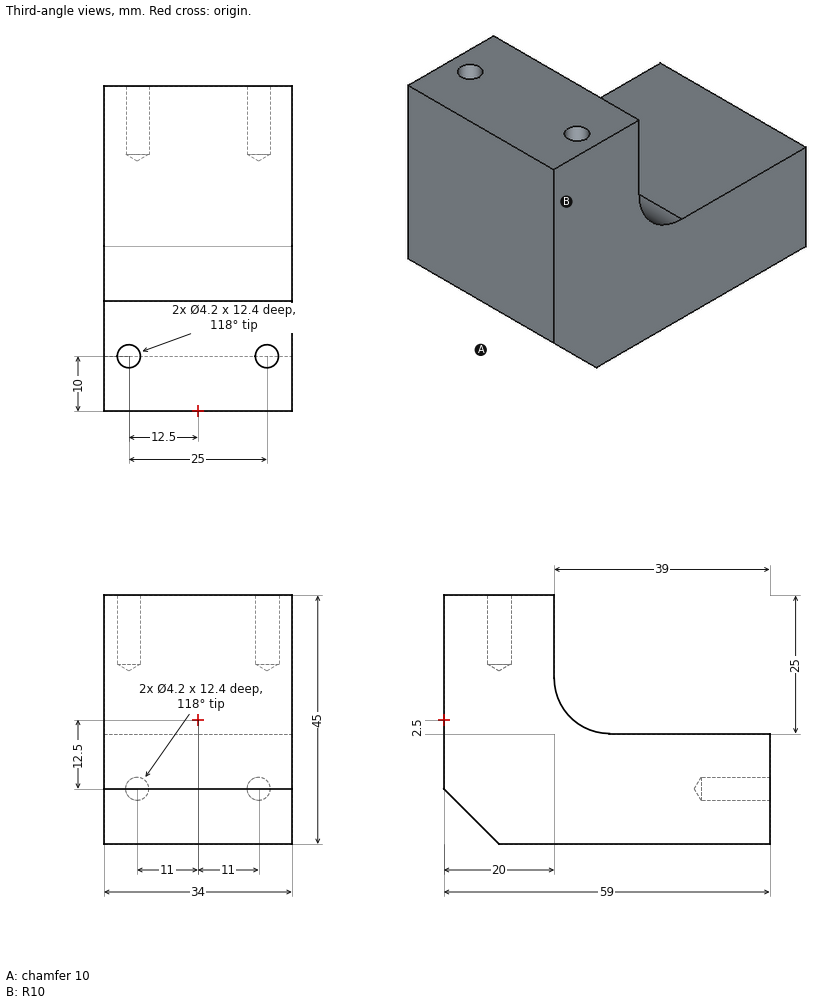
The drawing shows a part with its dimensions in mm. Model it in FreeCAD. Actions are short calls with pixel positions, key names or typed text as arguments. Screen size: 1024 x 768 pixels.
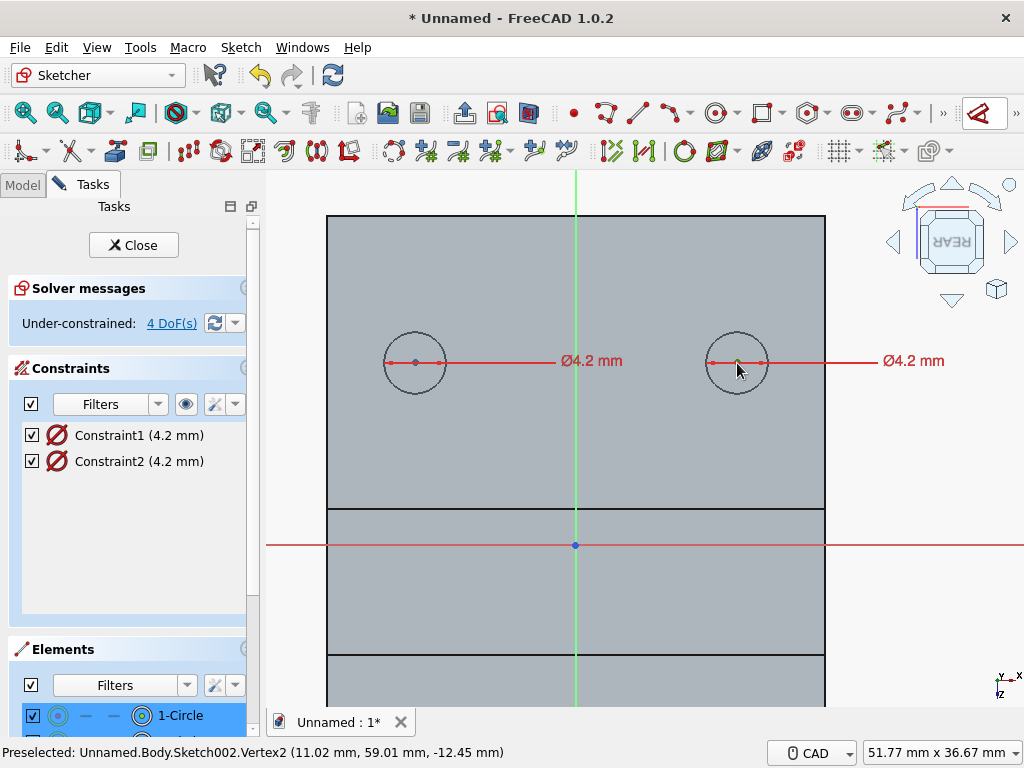
key(h)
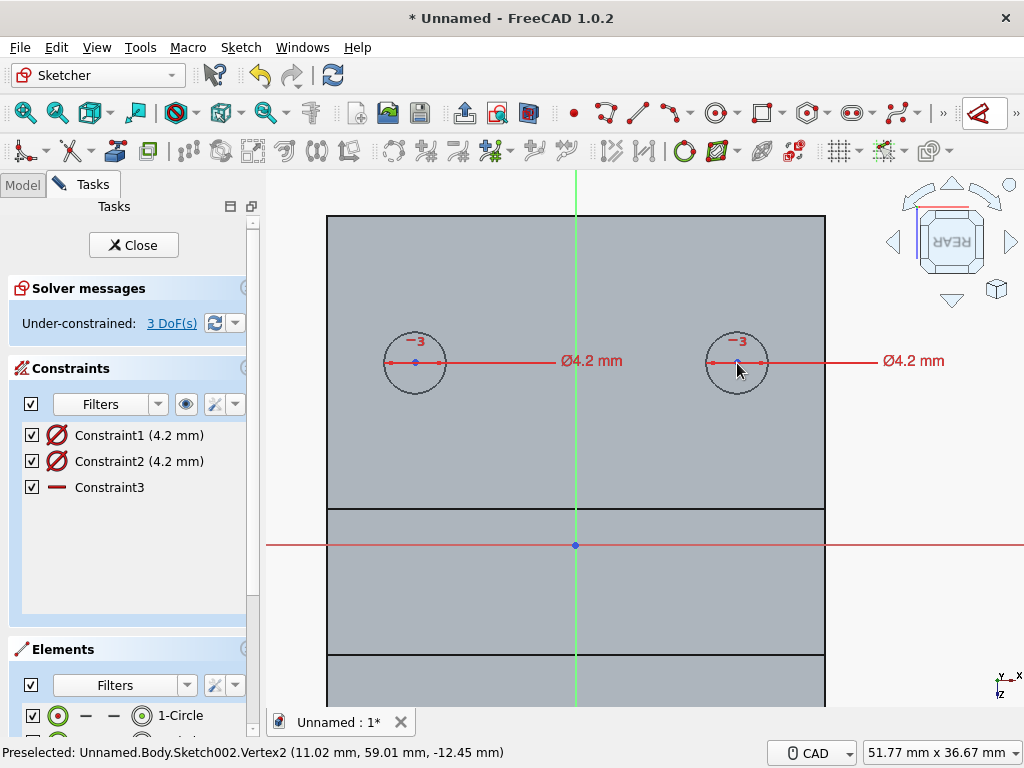
click(415, 363)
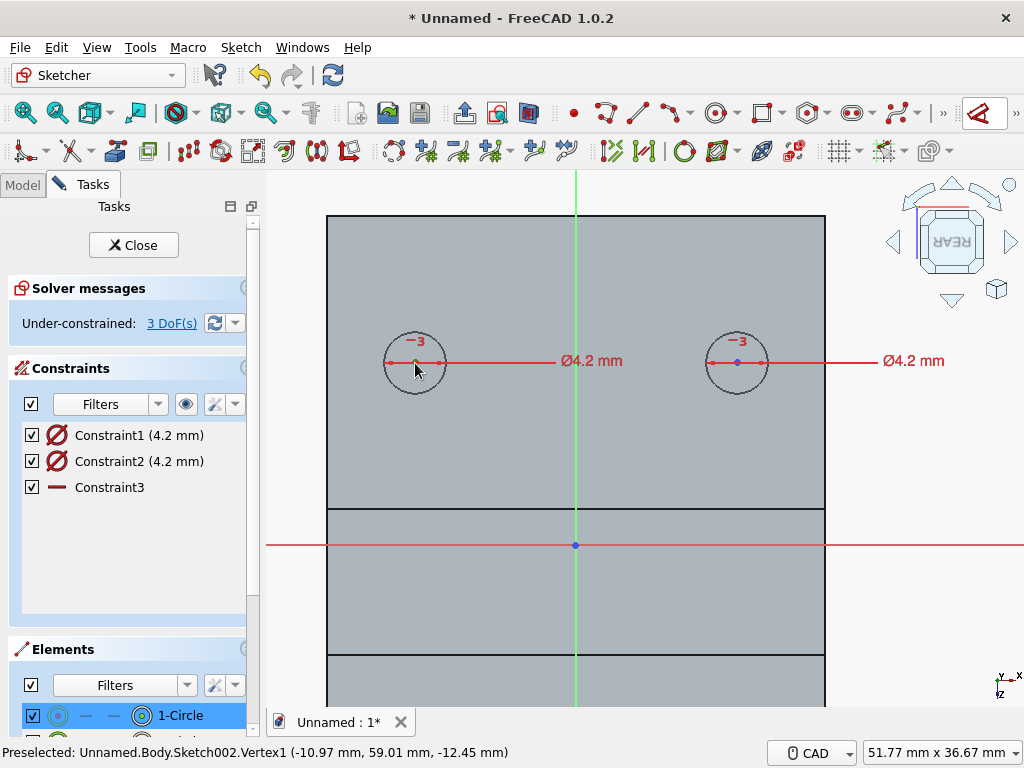
click(1002, 114)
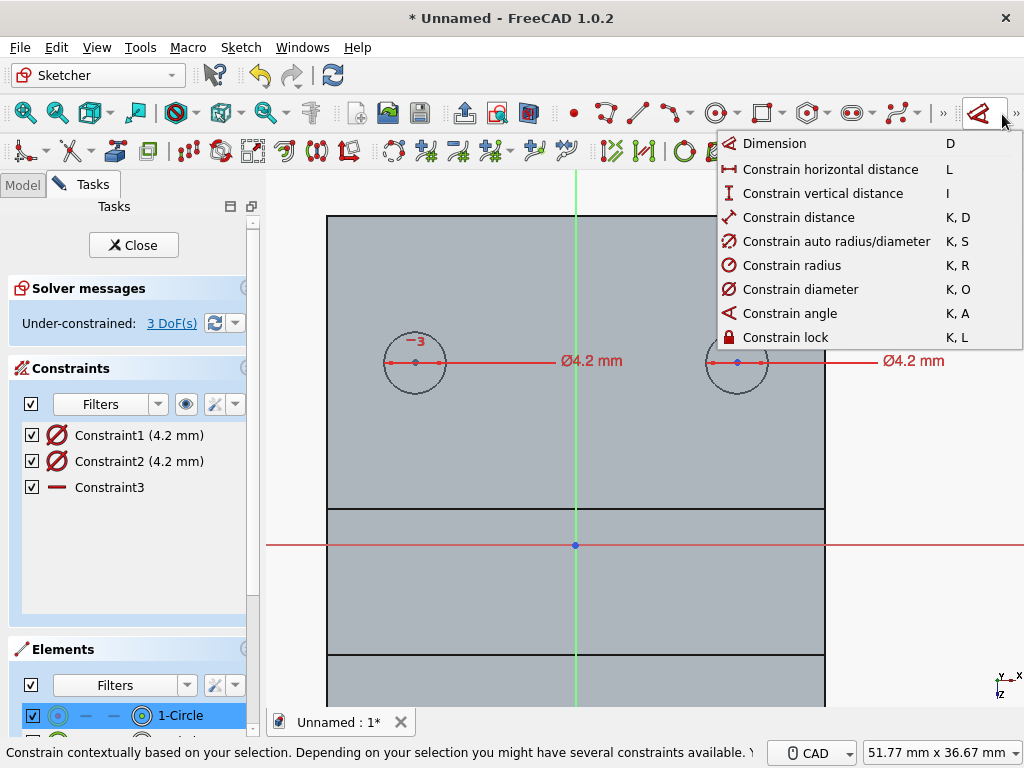
click(870, 169)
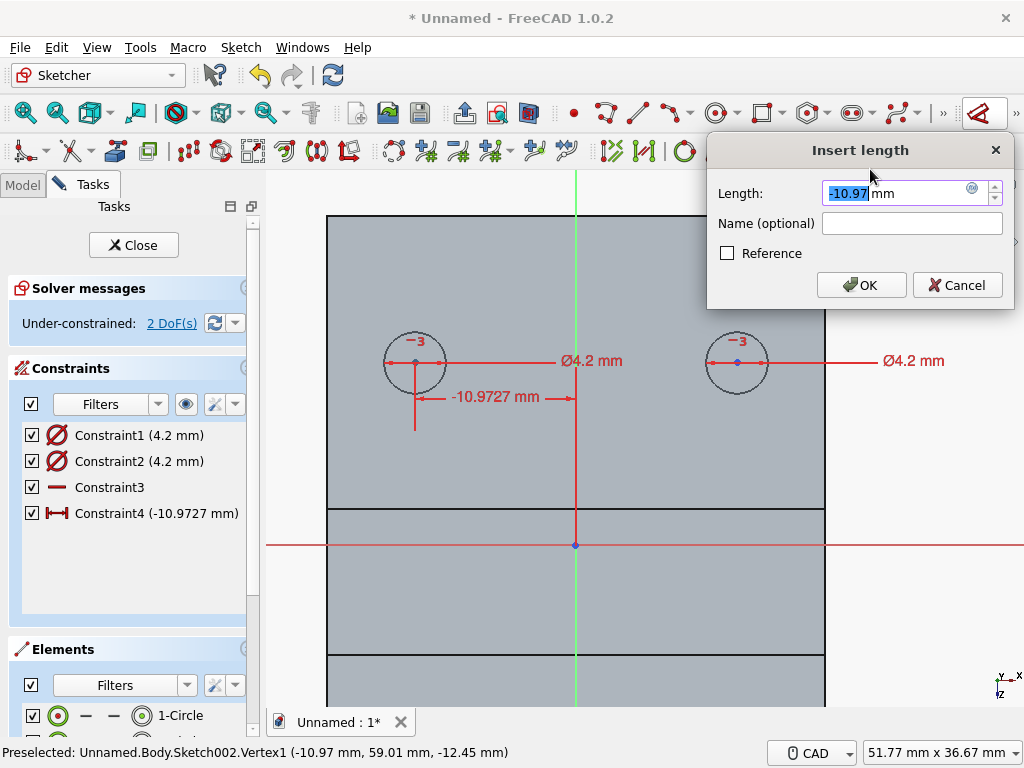
text(-11)
key(Return)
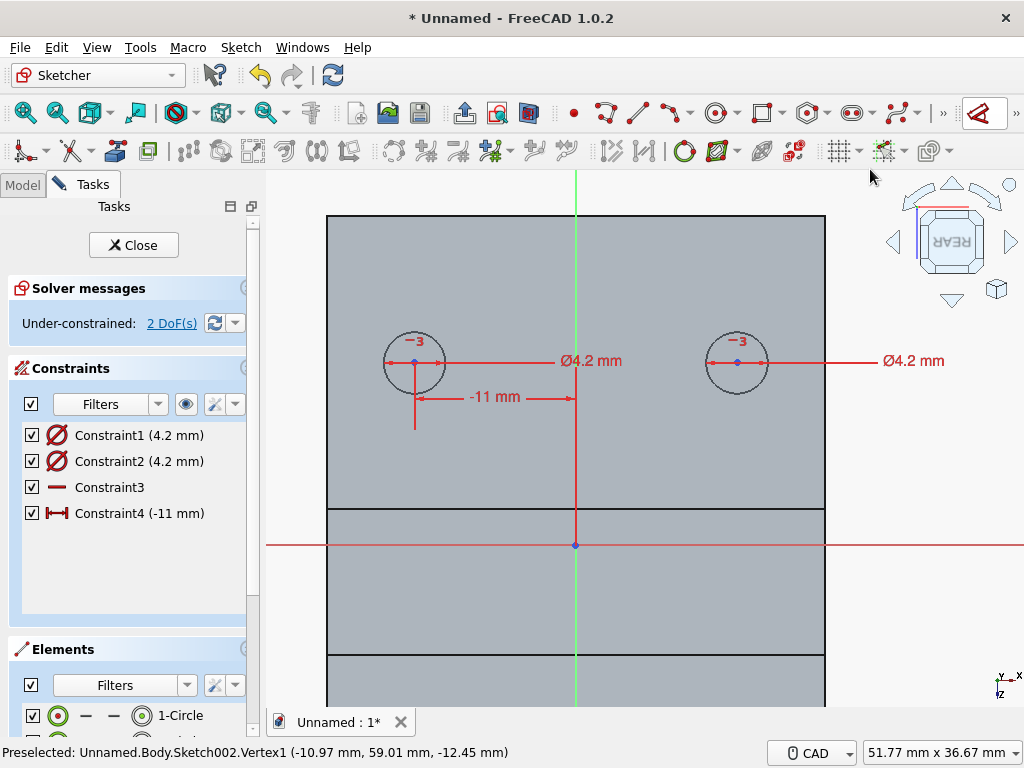
click(737, 363)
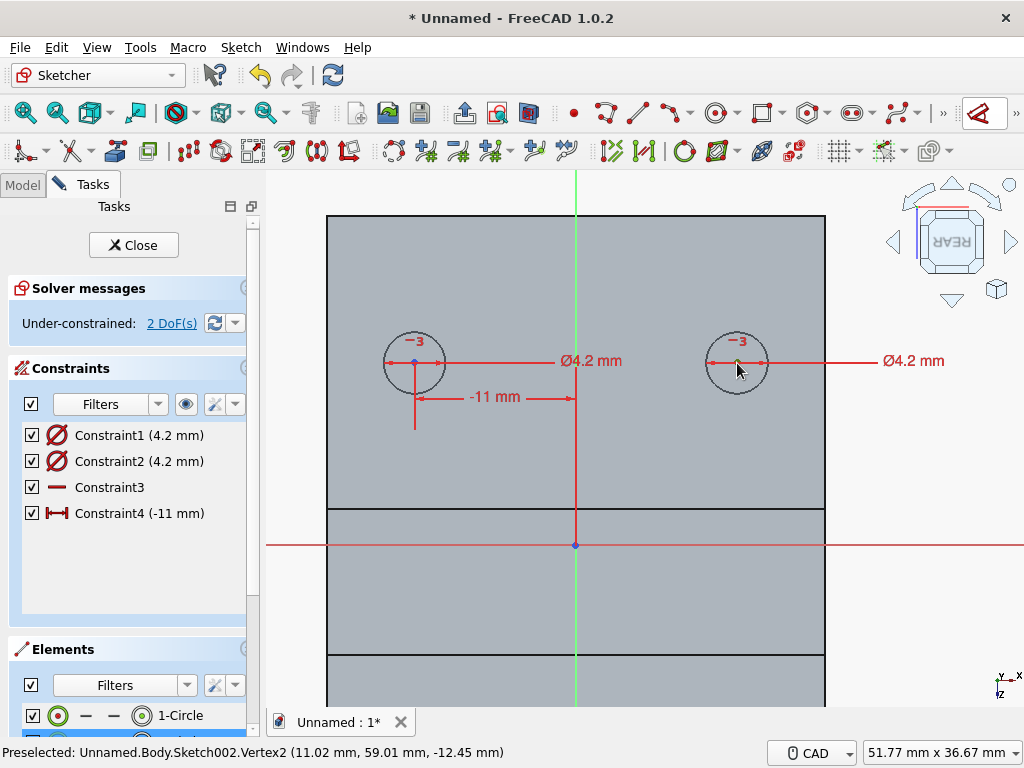
key(l)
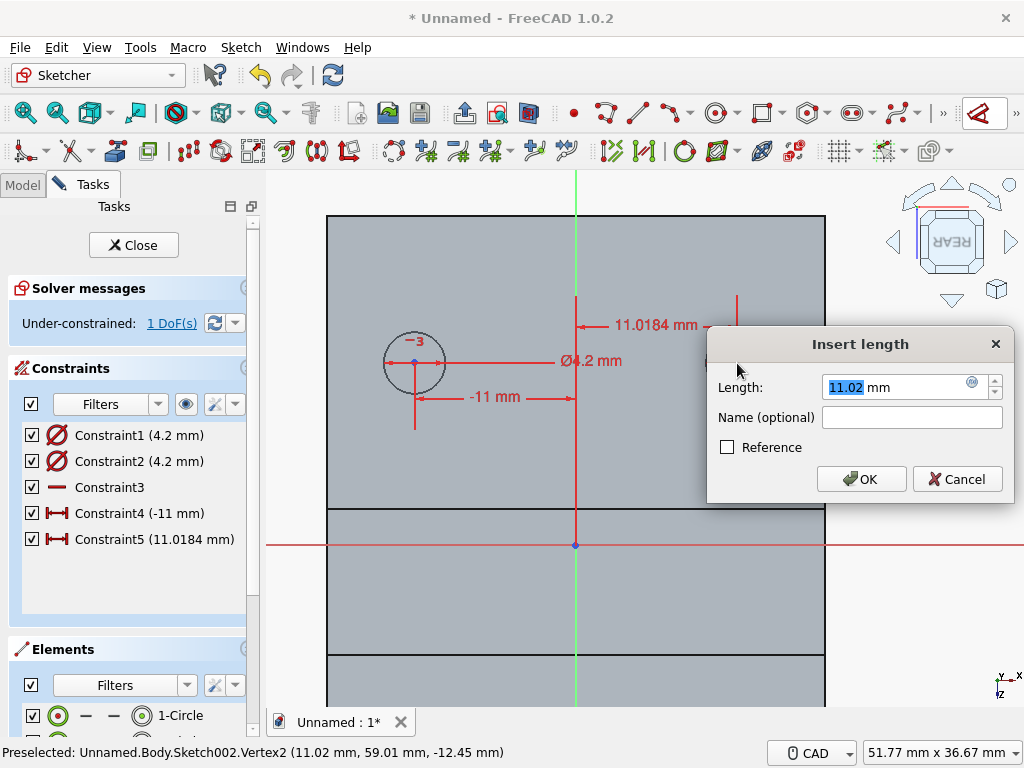
text(11)
key(Return)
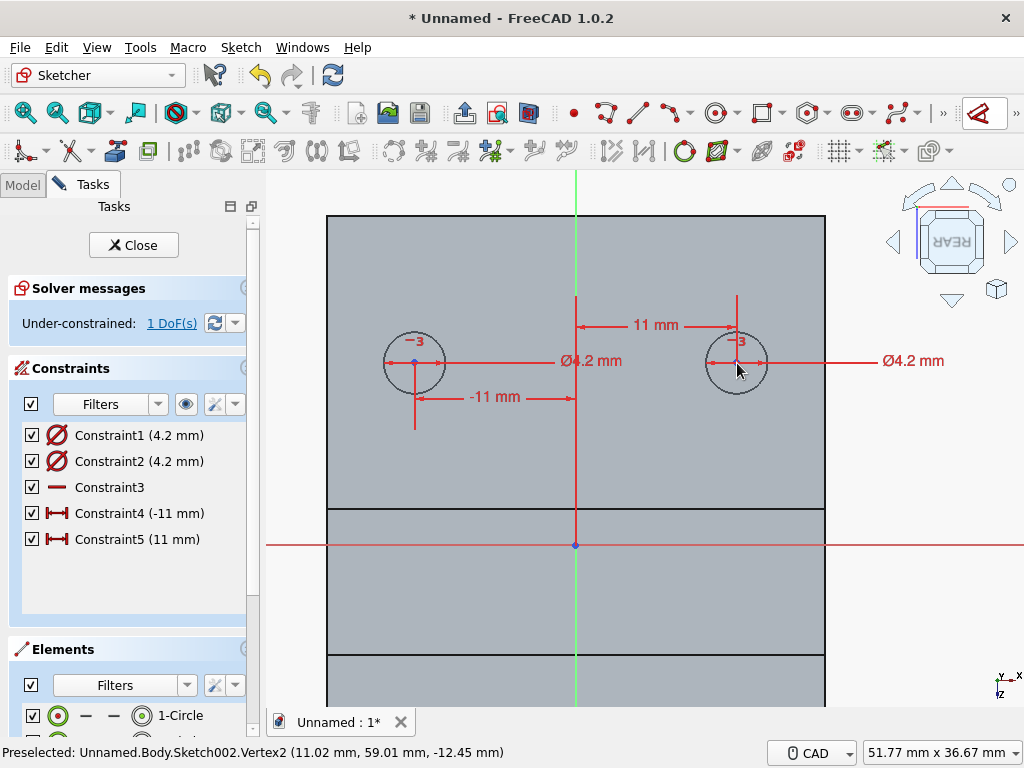
click(415, 363)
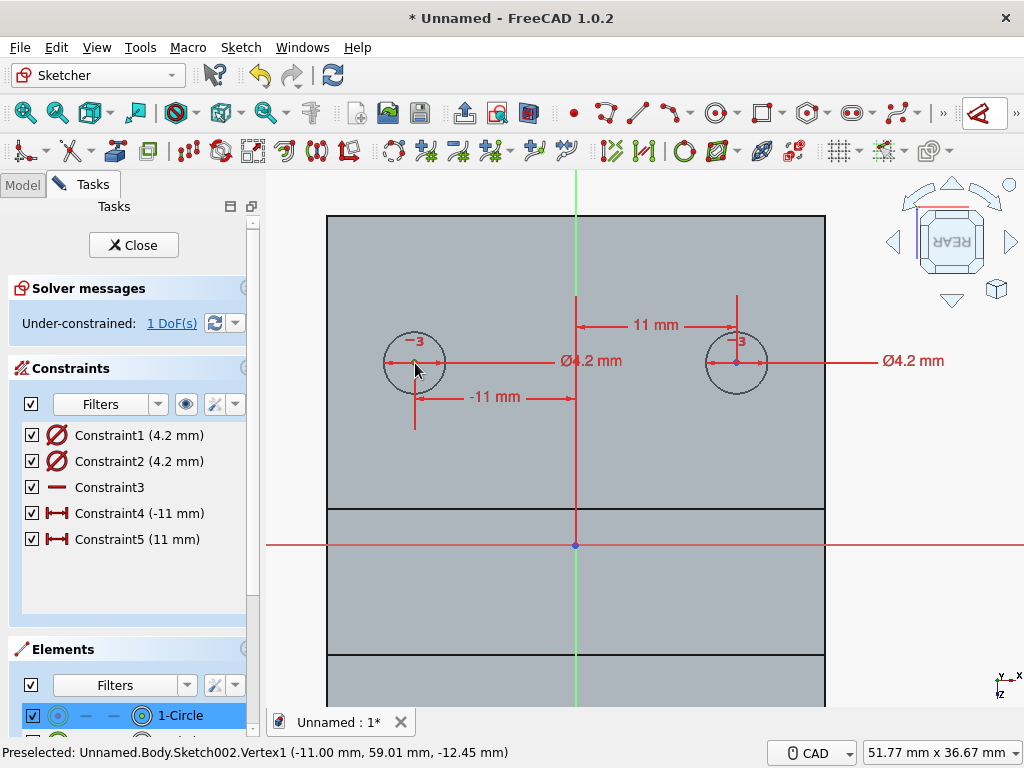
key(i)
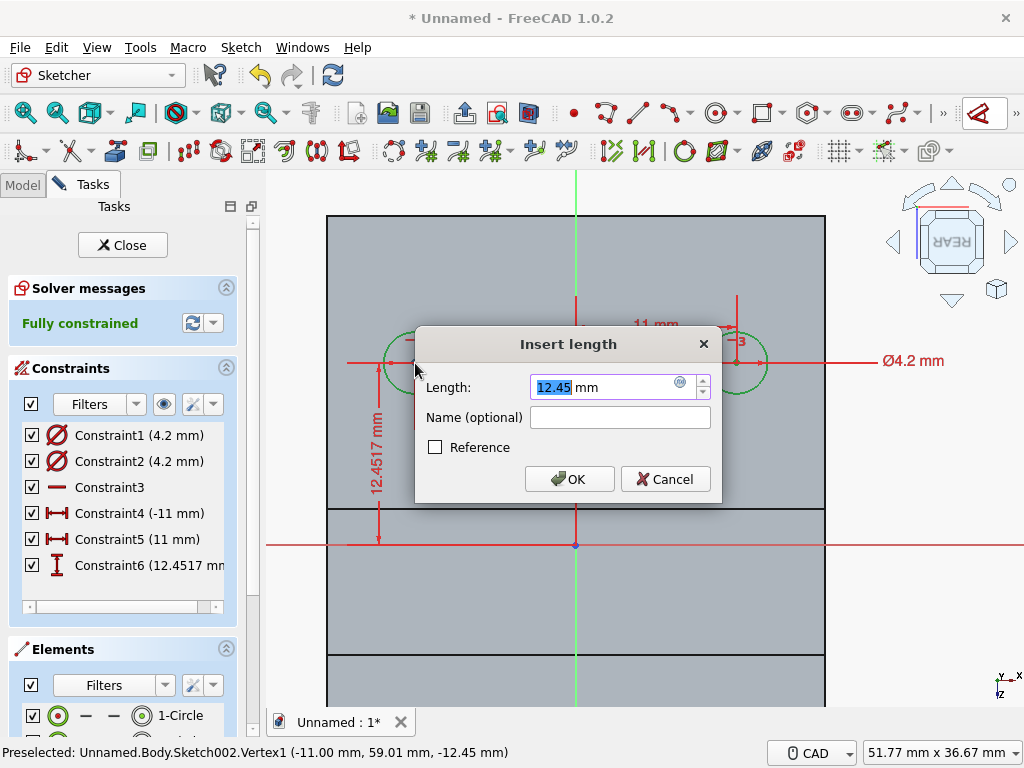
text(12.5)
key(Return)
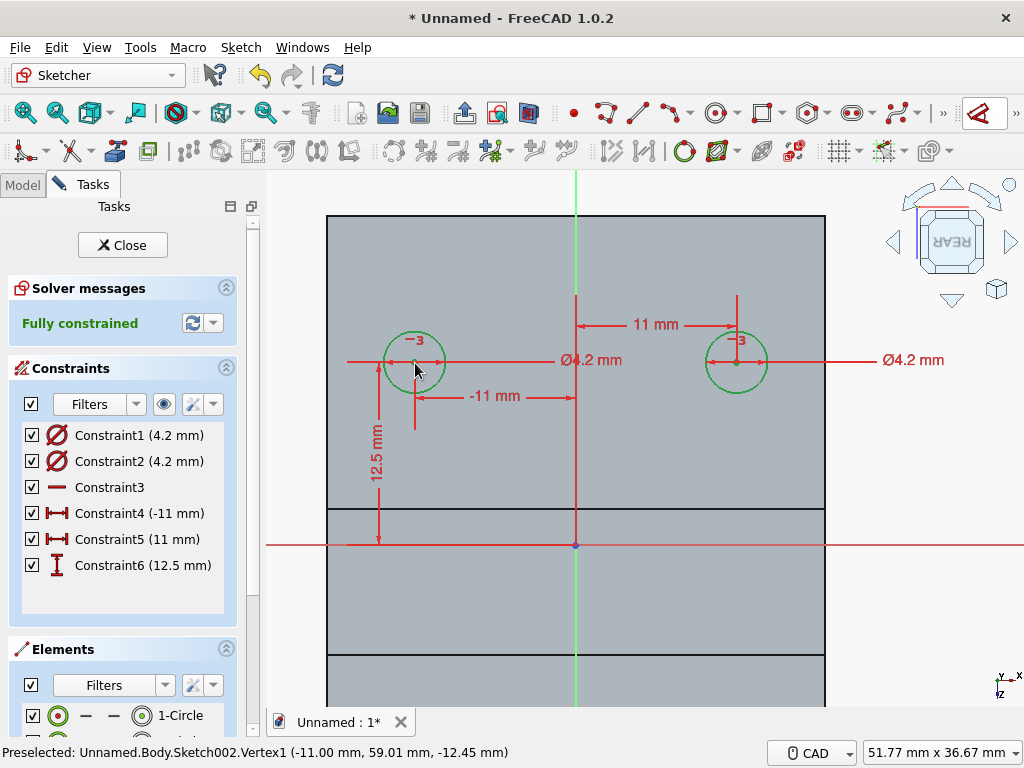
click(123, 245)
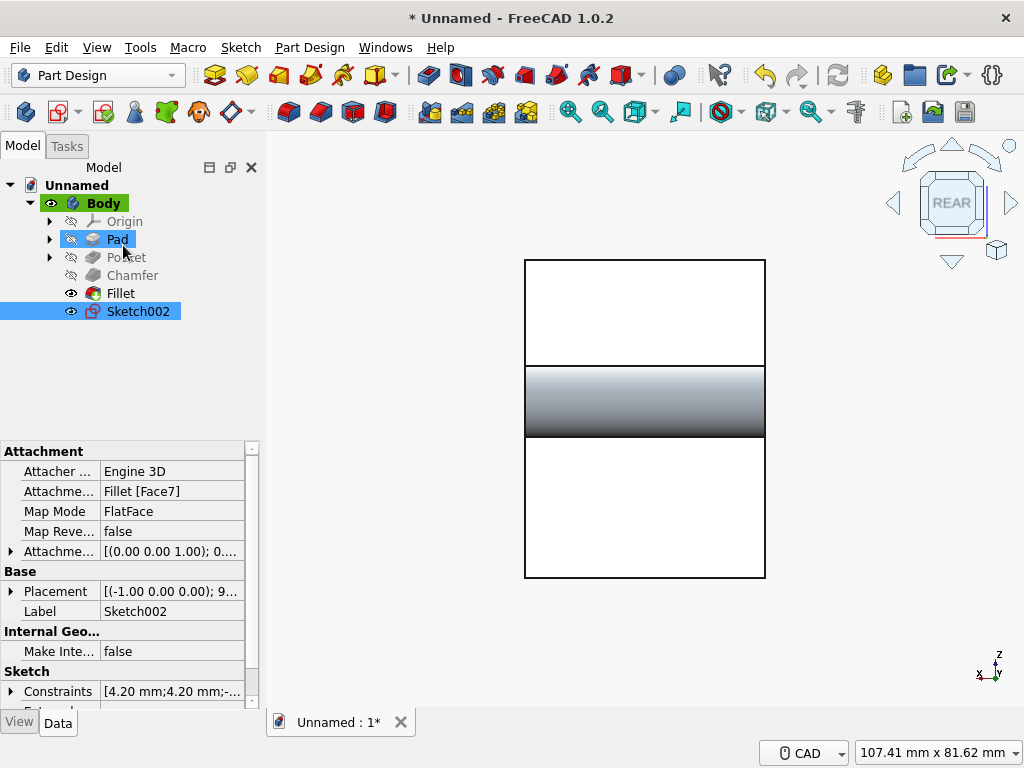
click(462, 76)